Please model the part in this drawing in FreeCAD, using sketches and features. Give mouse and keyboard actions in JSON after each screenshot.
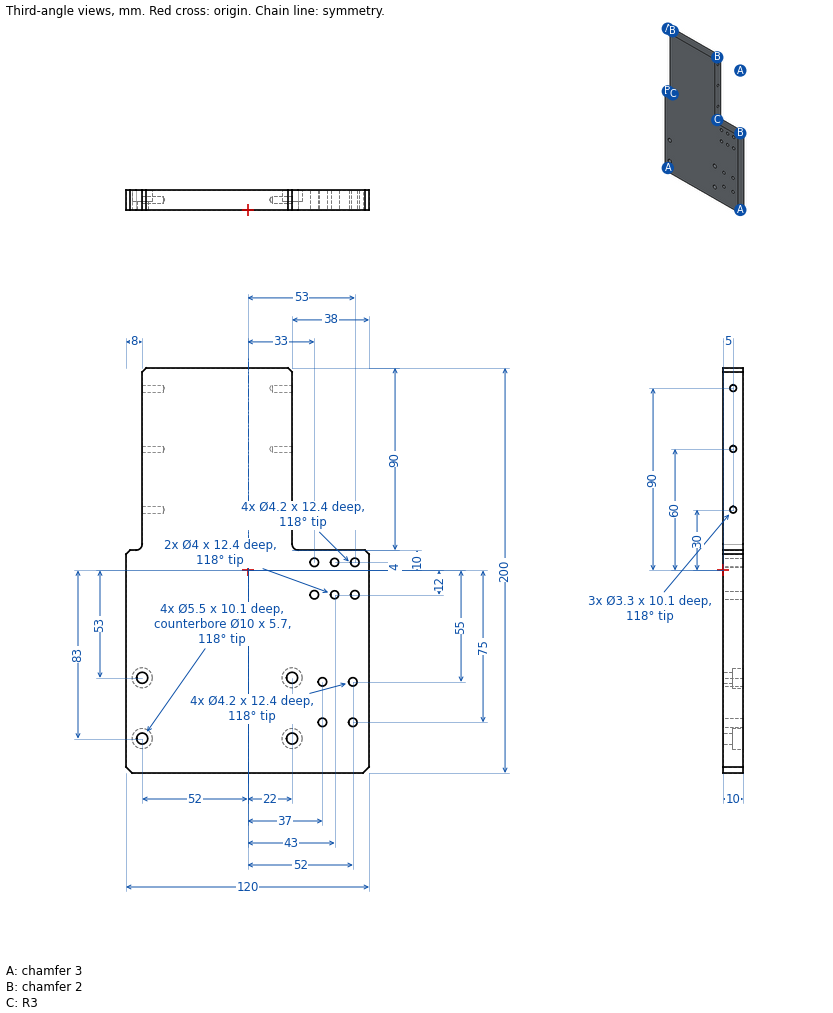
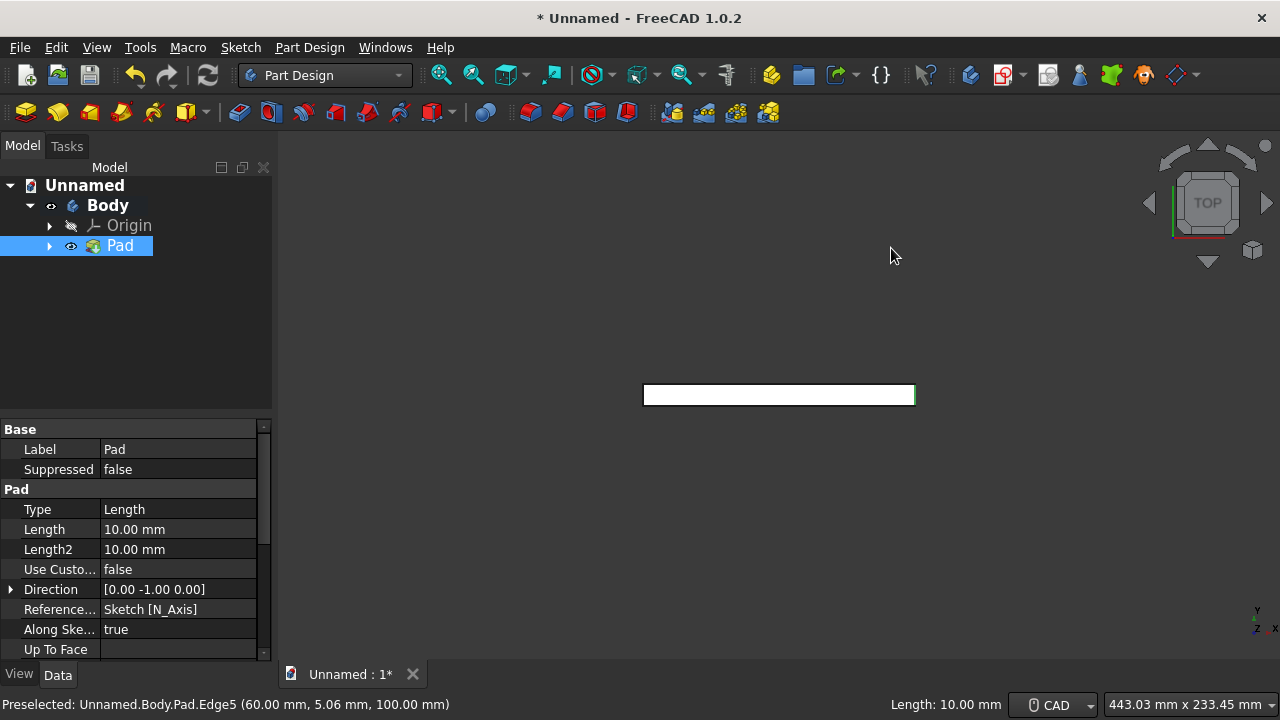
{"action": "left_click", "coordinate": [643, 394], "text": "ctrl"}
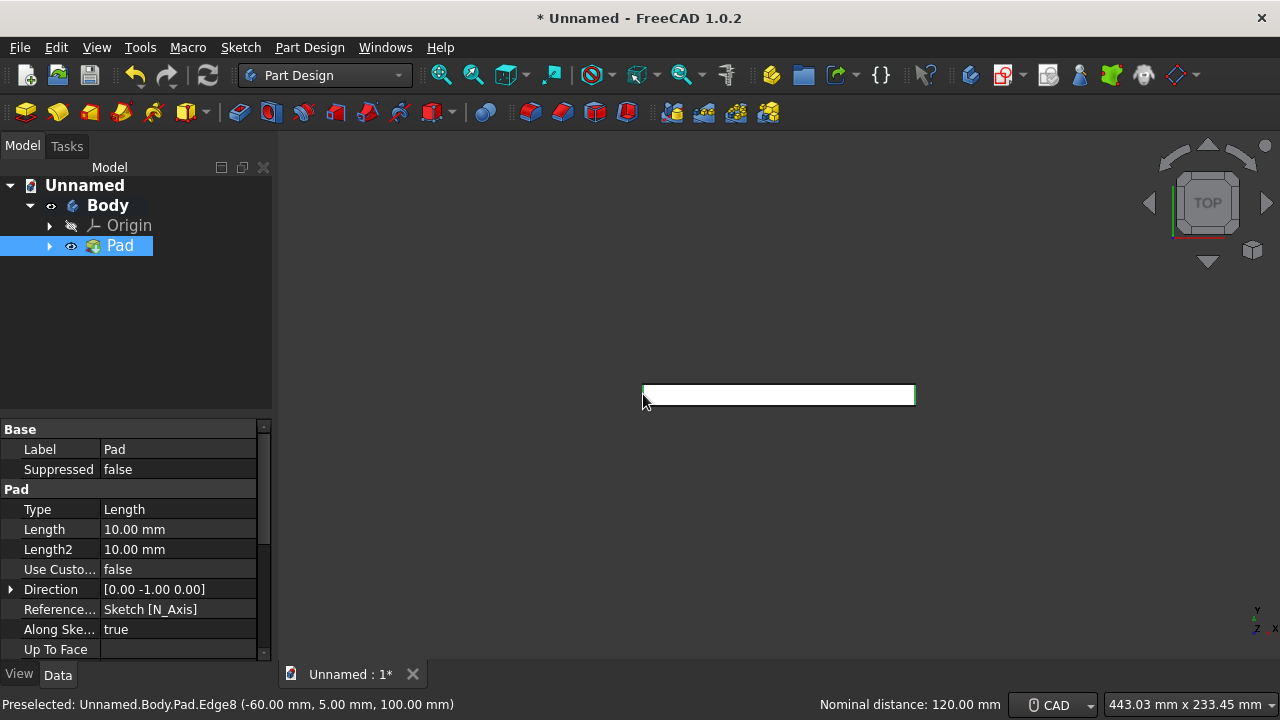
{"action": "key", "text": "1"}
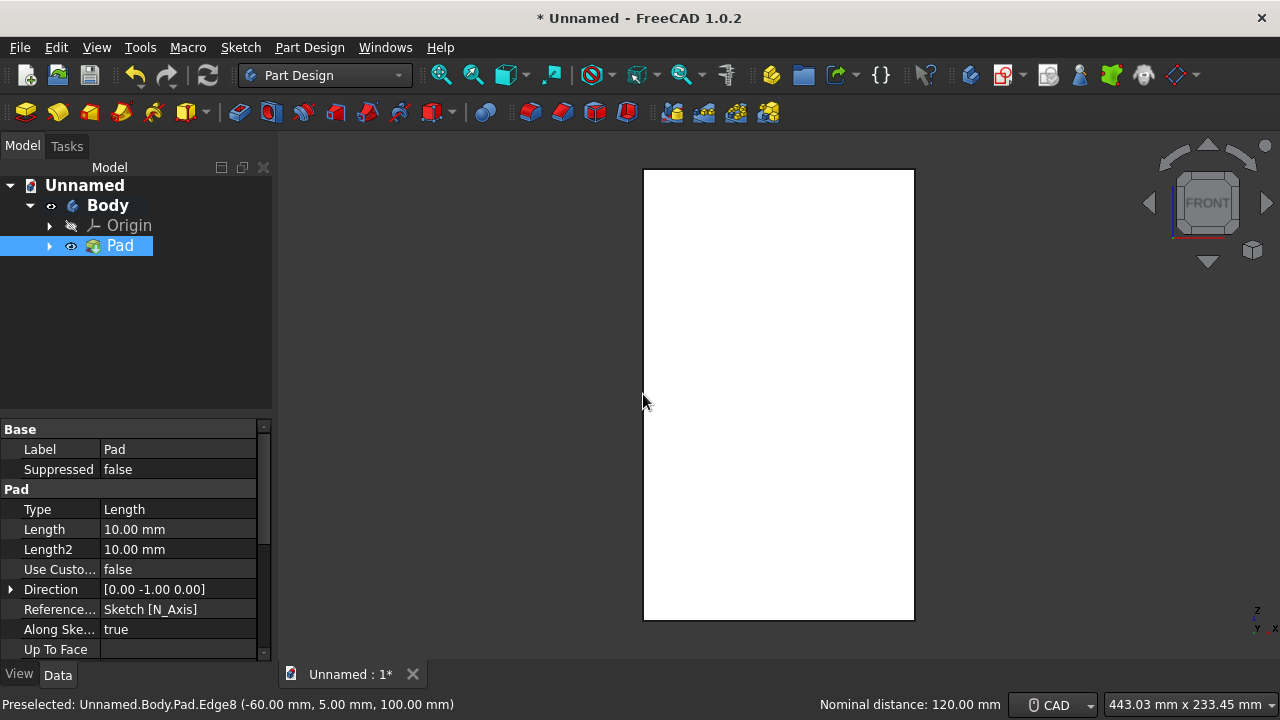
{"action": "key", "text": "3"}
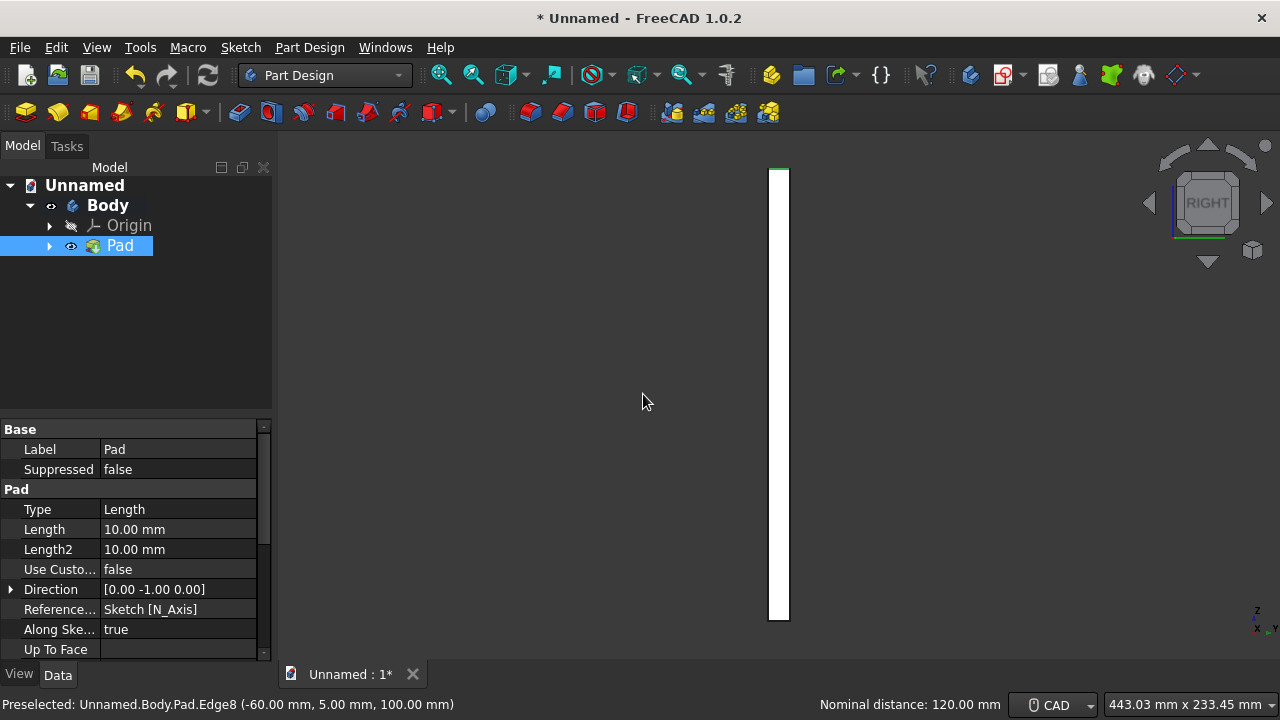
{"action": "left_click", "coordinate": [779, 620], "text": "ctrl"}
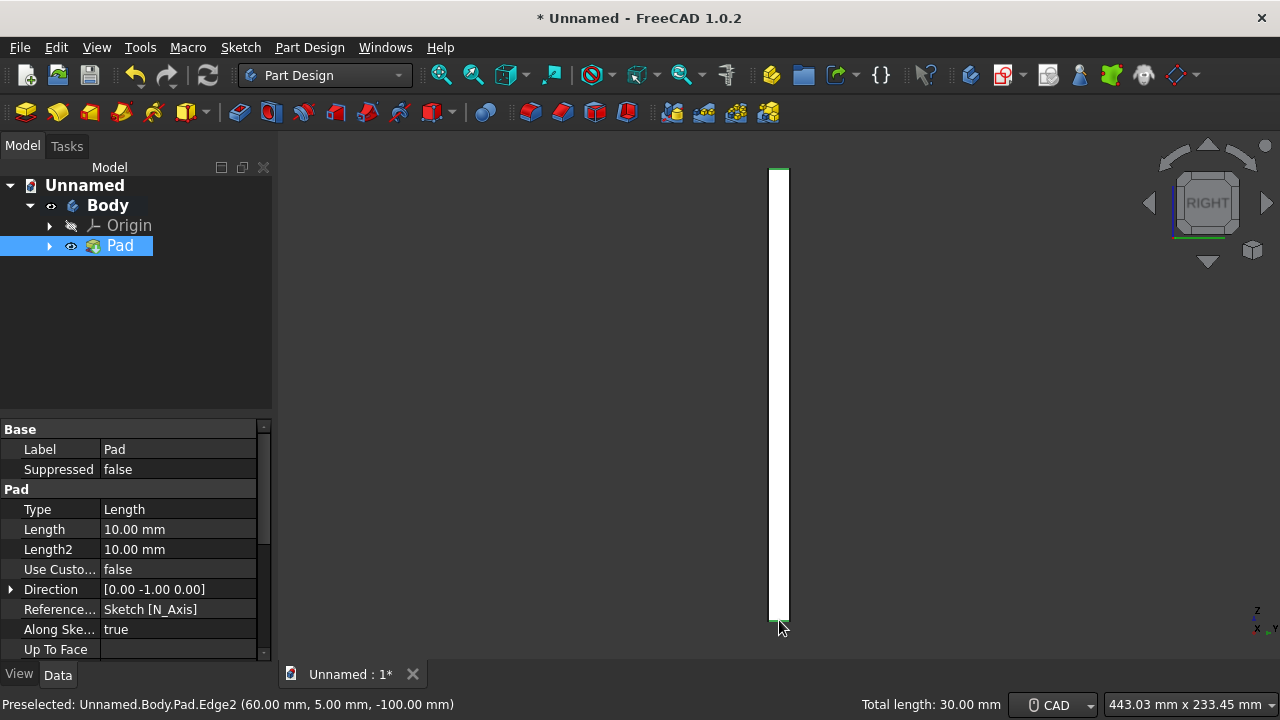
{"action": "key", "text": "5"}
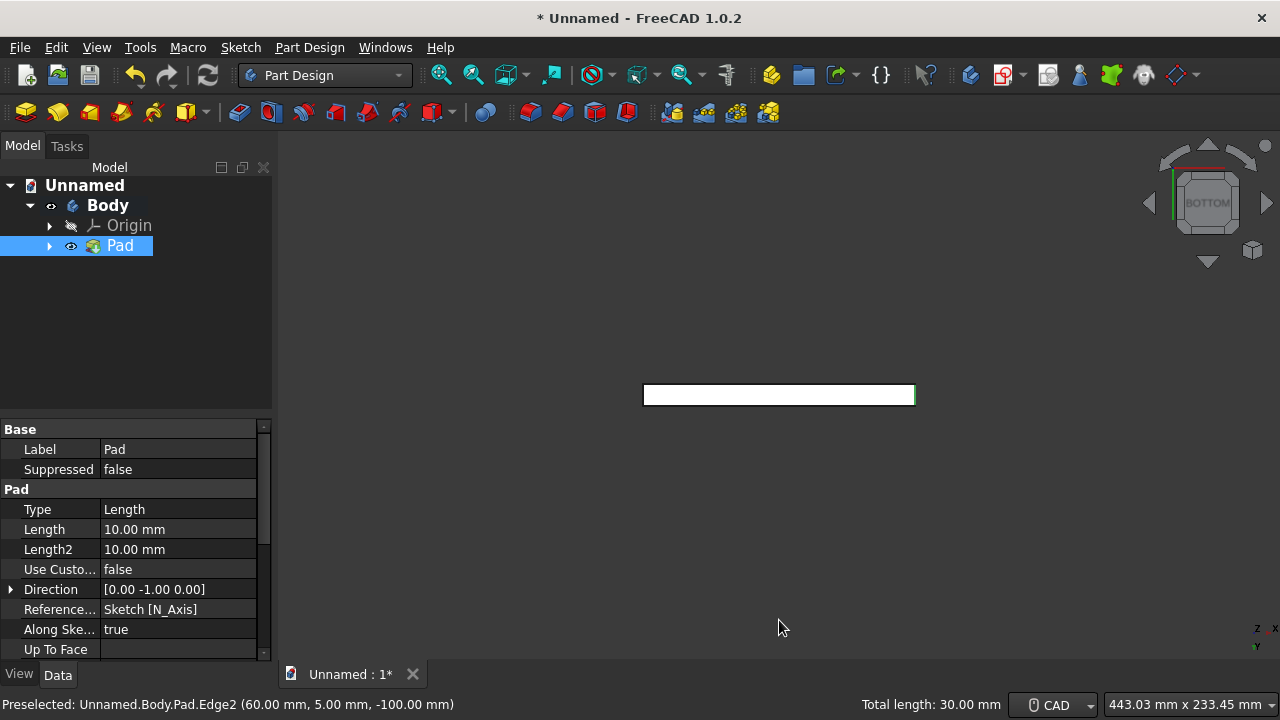
{"action": "left_click", "coordinate": [442, 76]}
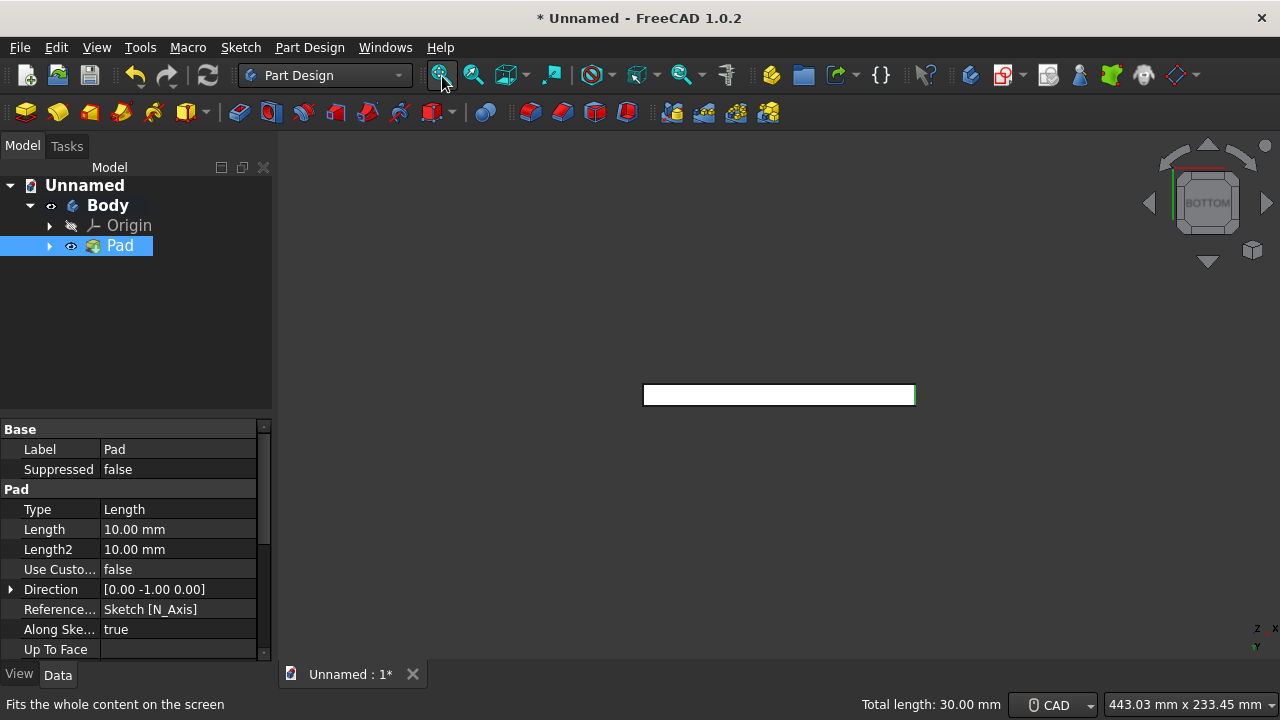
{"action": "left_click", "coordinate": [643, 394], "text": "ctrl"}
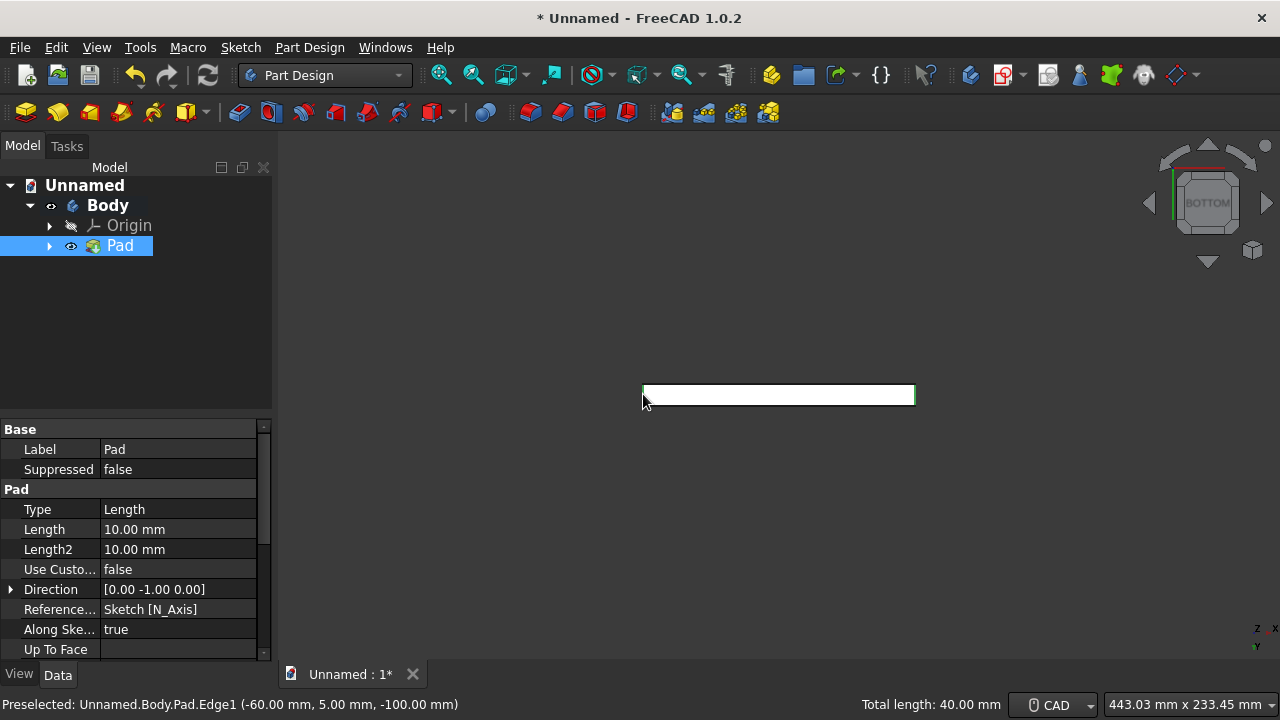
{"action": "left_click", "coordinate": [564, 112]}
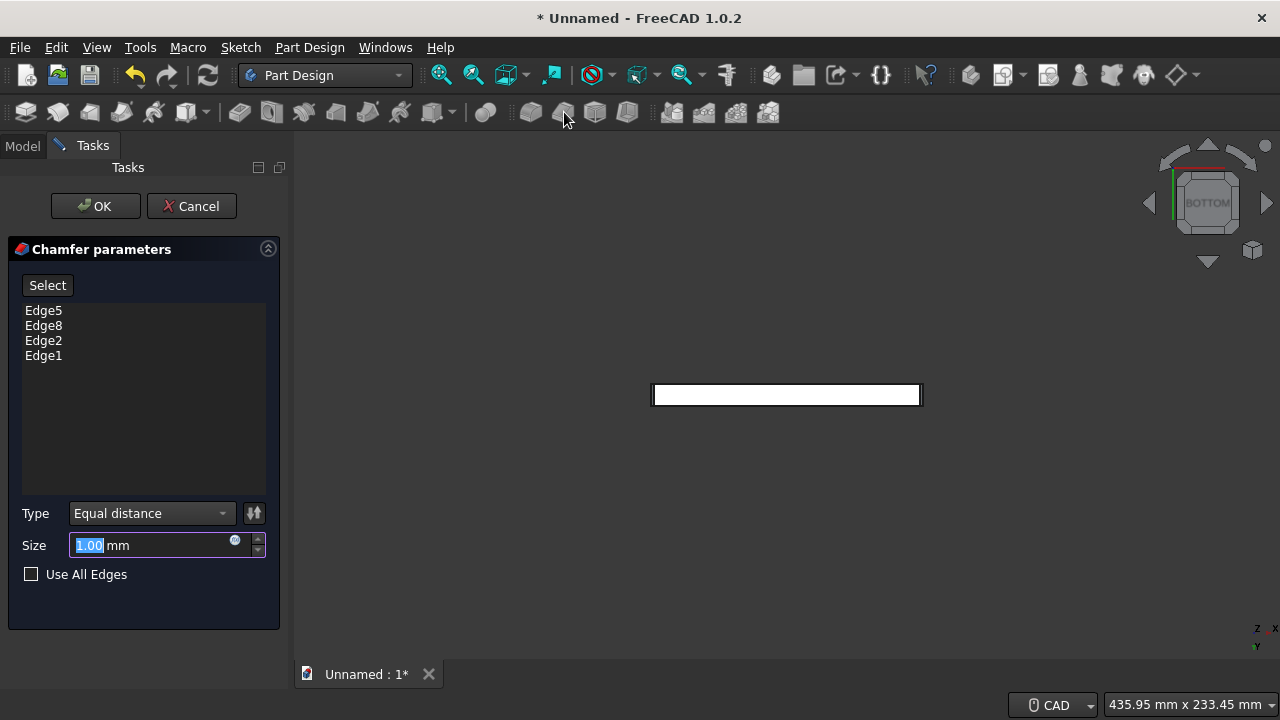
{"action": "type", "text": "3"}
{"action": "key", "text": "Tab"}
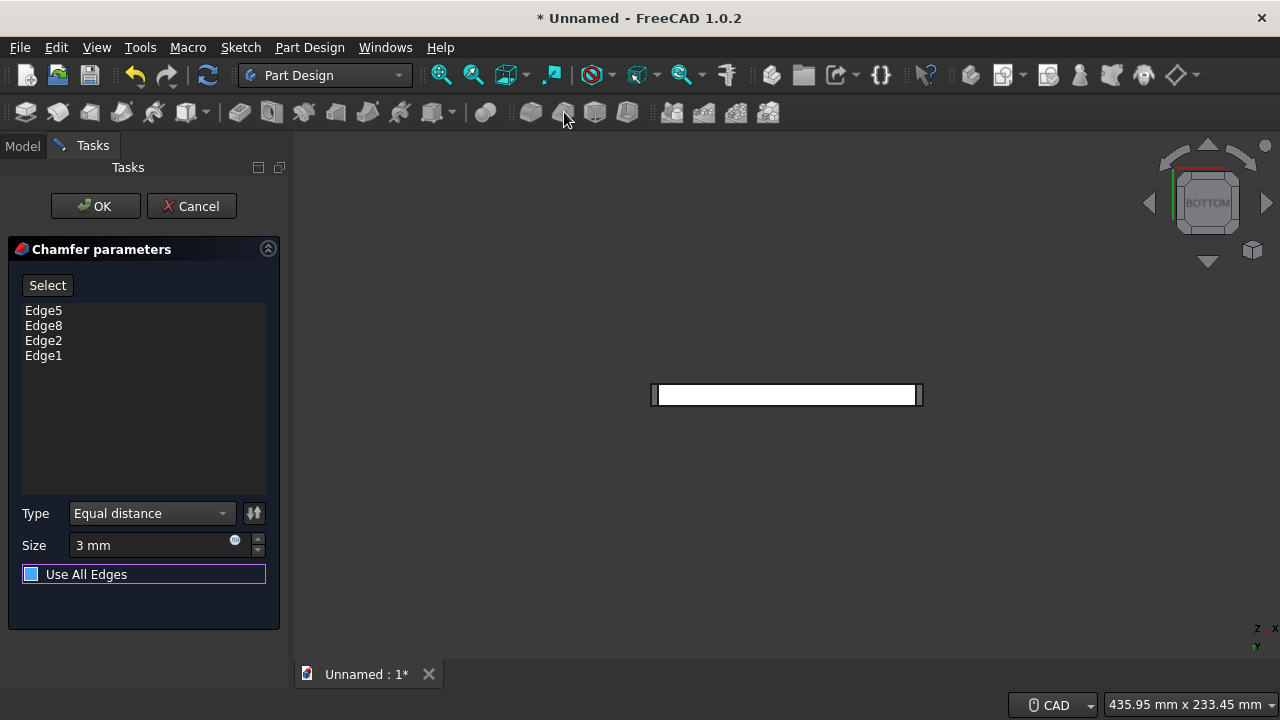
{"action": "left_click", "coordinate": [96, 206]}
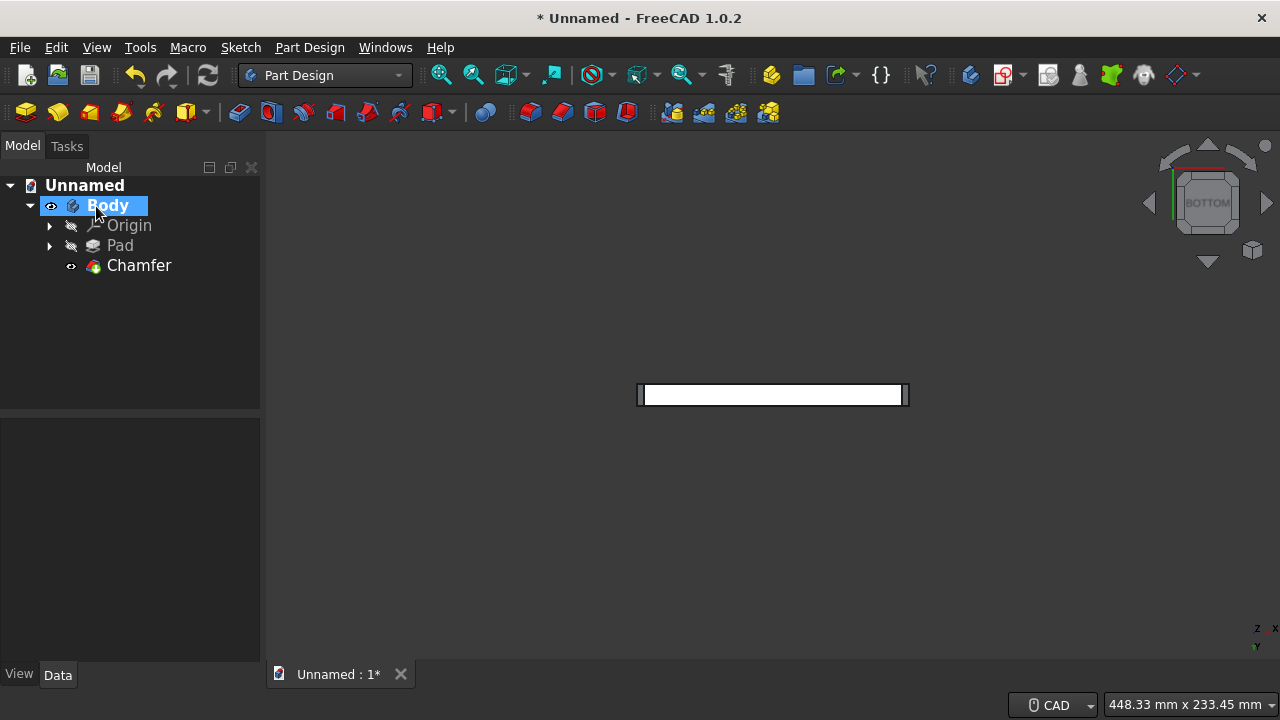
{"action": "left_click", "coordinate": [442, 76]}